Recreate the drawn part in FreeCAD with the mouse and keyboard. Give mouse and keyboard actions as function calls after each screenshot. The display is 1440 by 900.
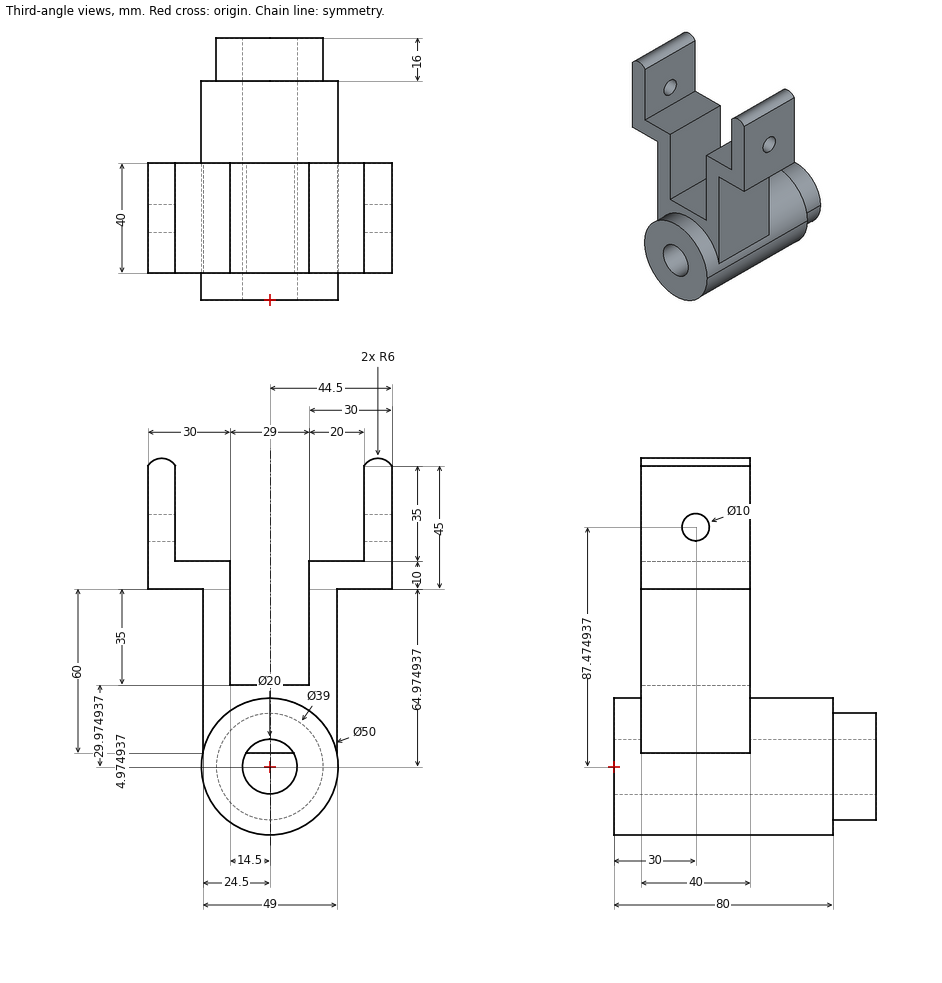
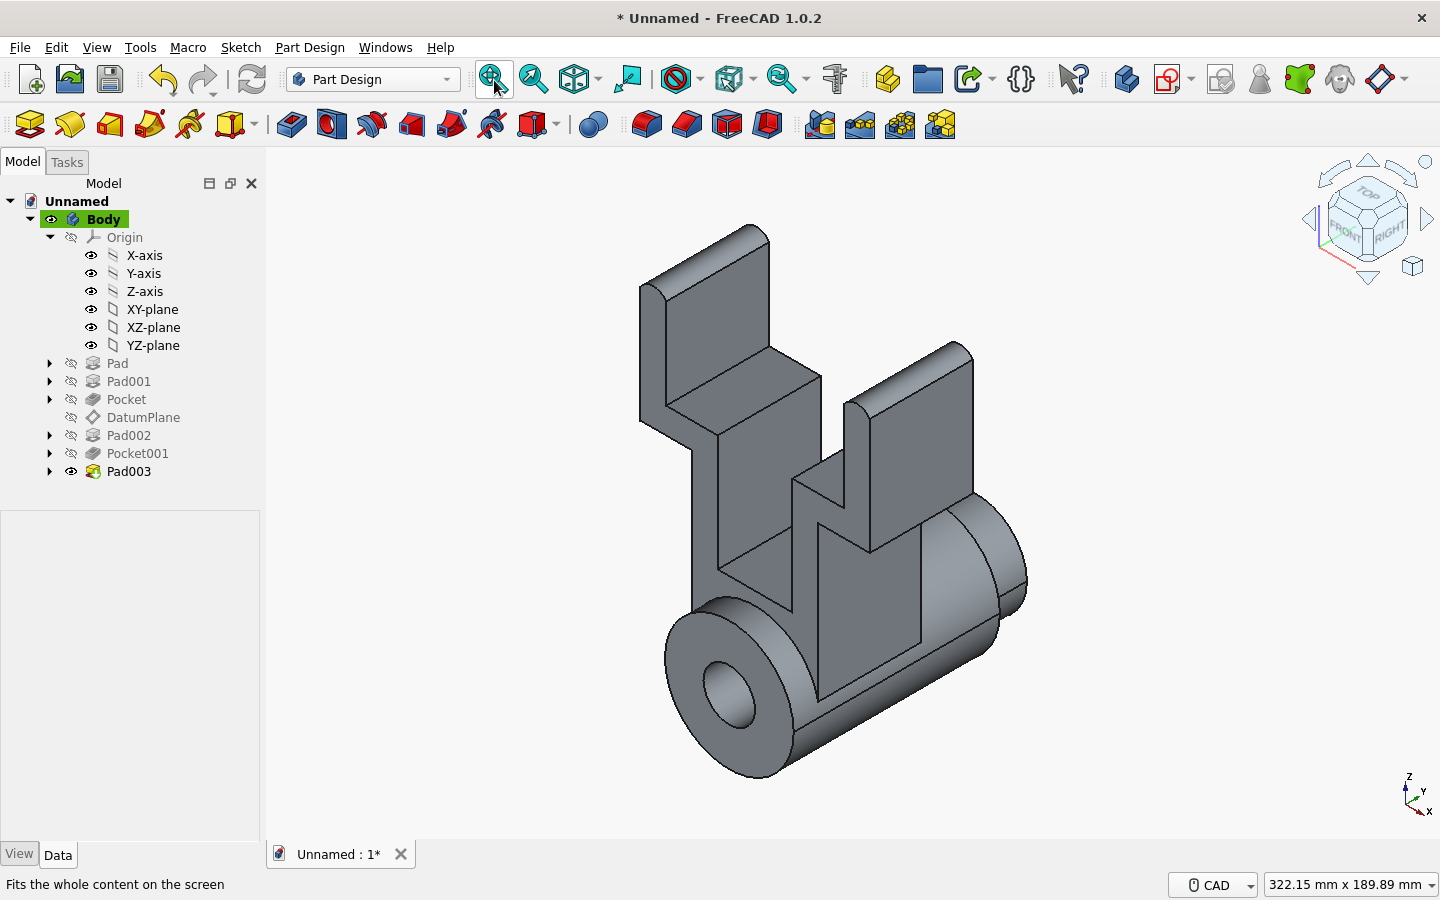
click(921, 455)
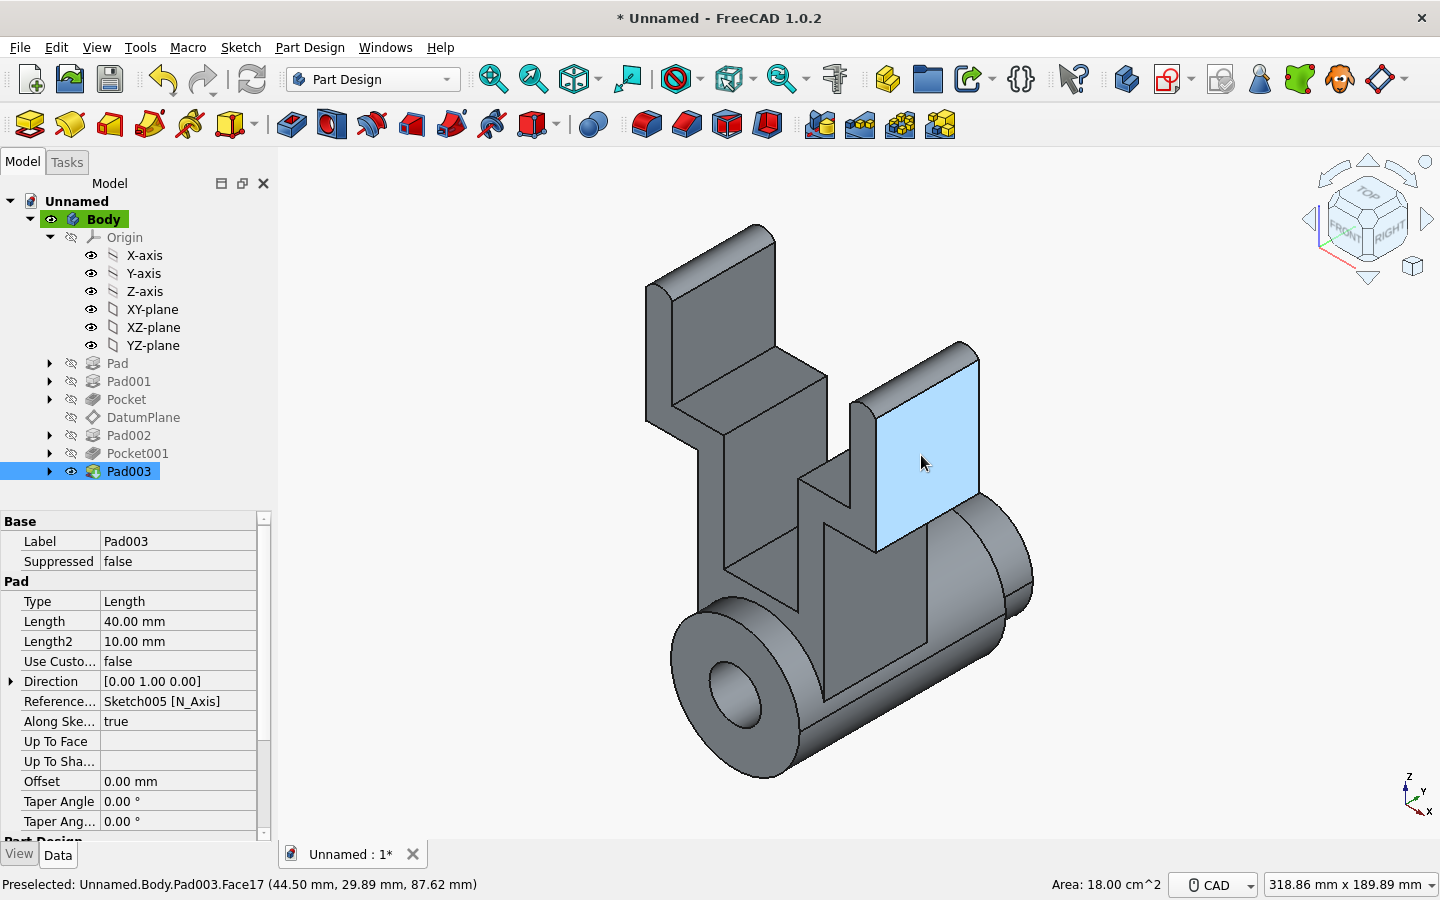
click(1168, 80)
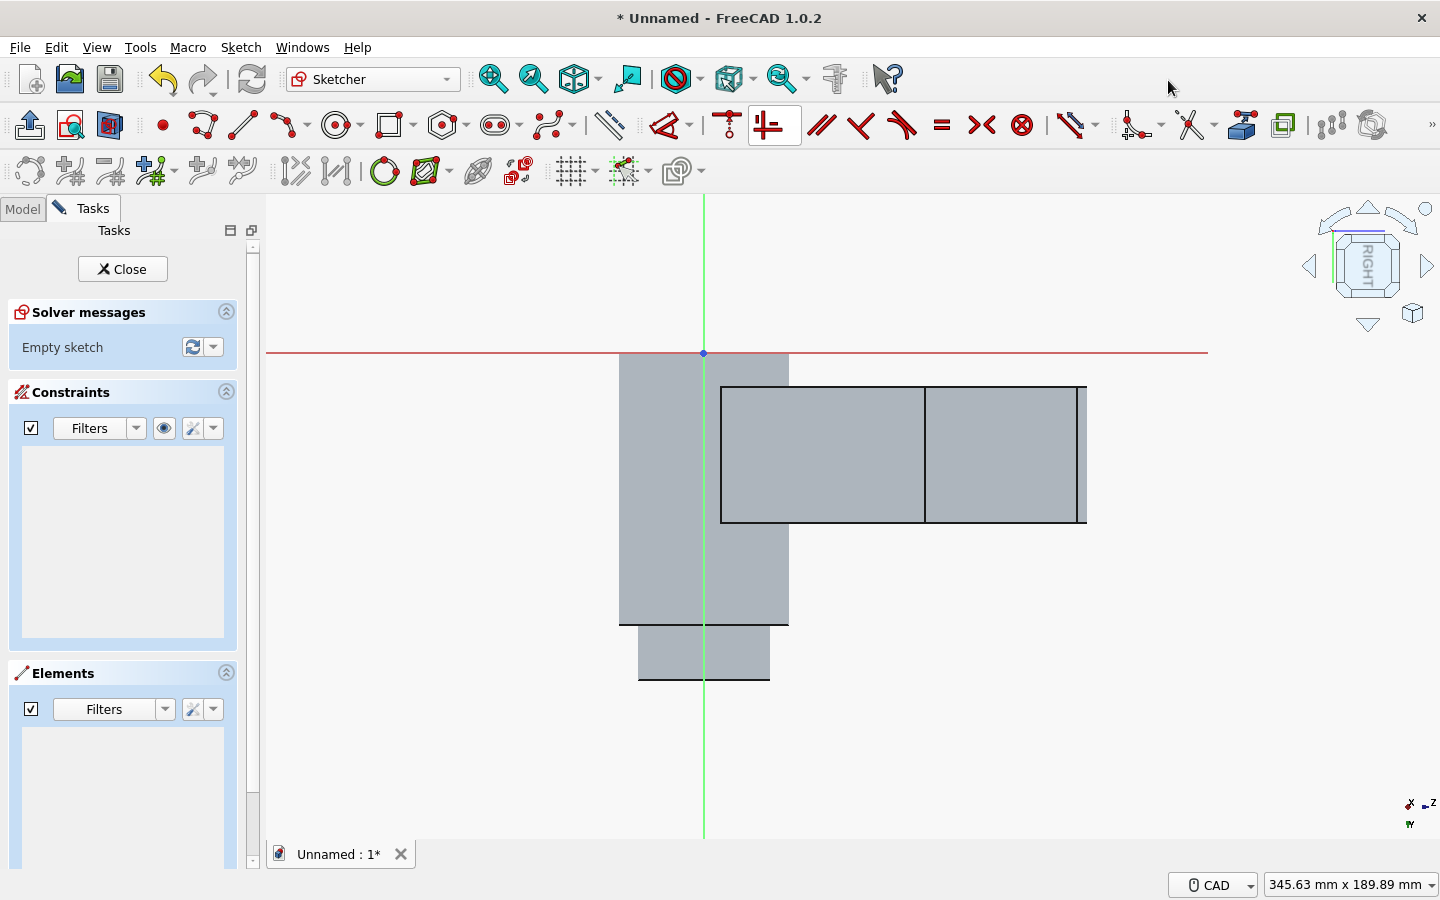
scroll(1018, 450, up, 13)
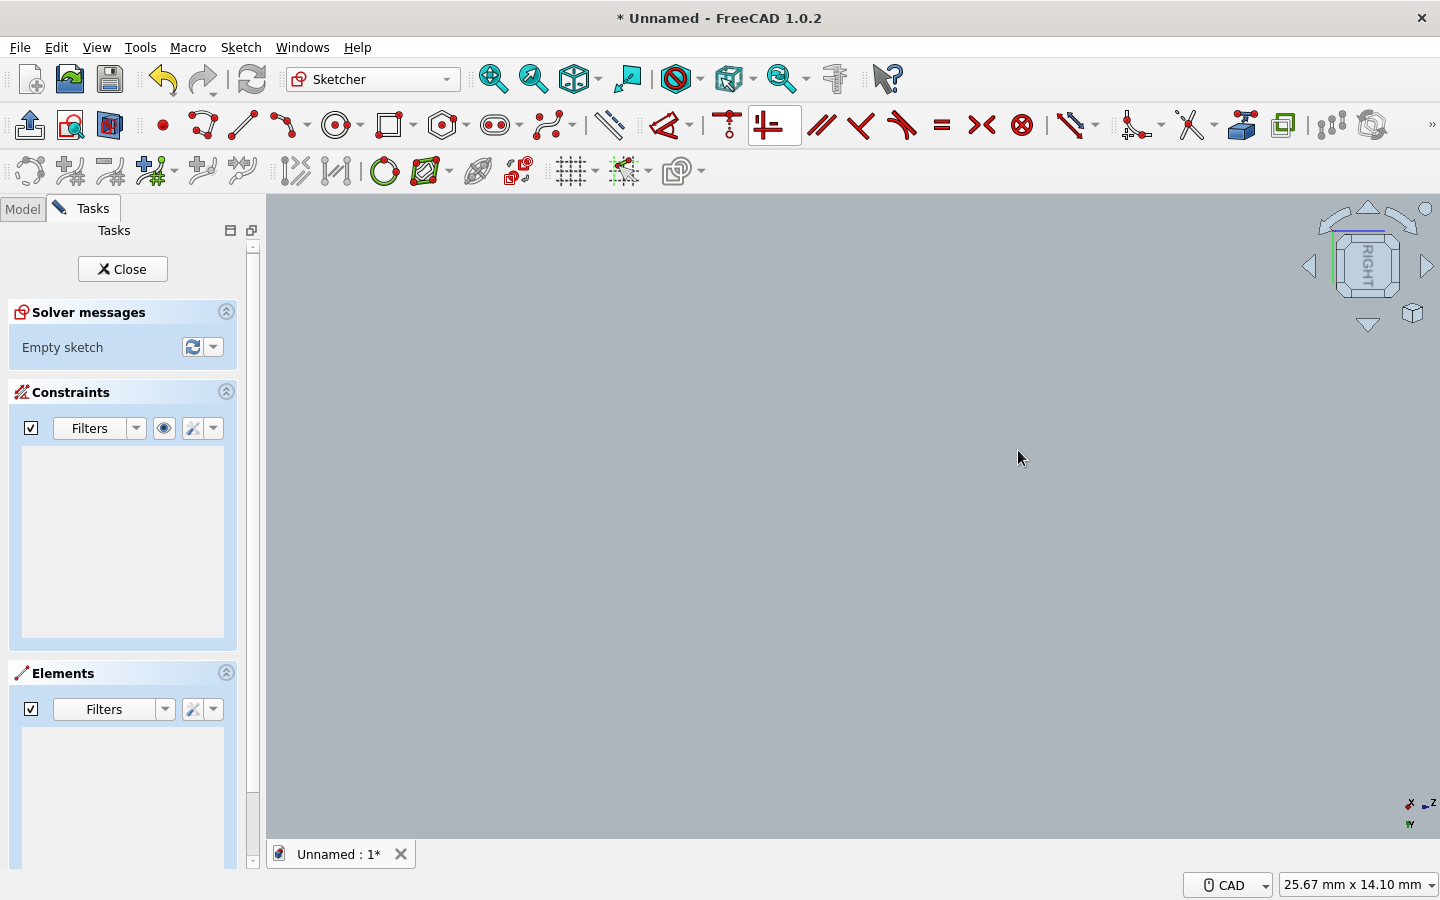
click(336, 126)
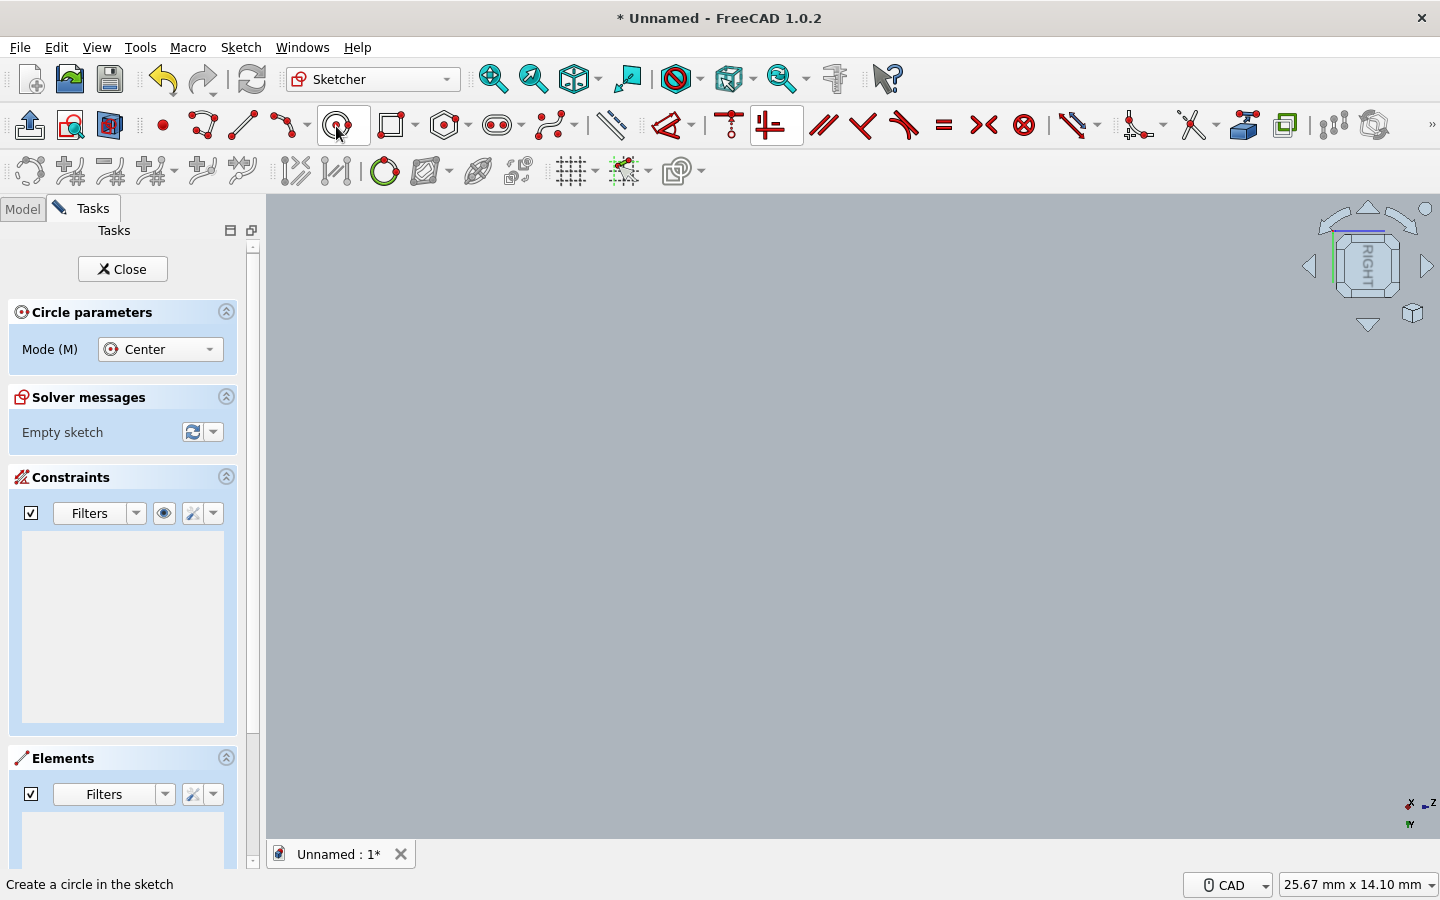
click(782, 517)
click(944, 356)
key(Escape)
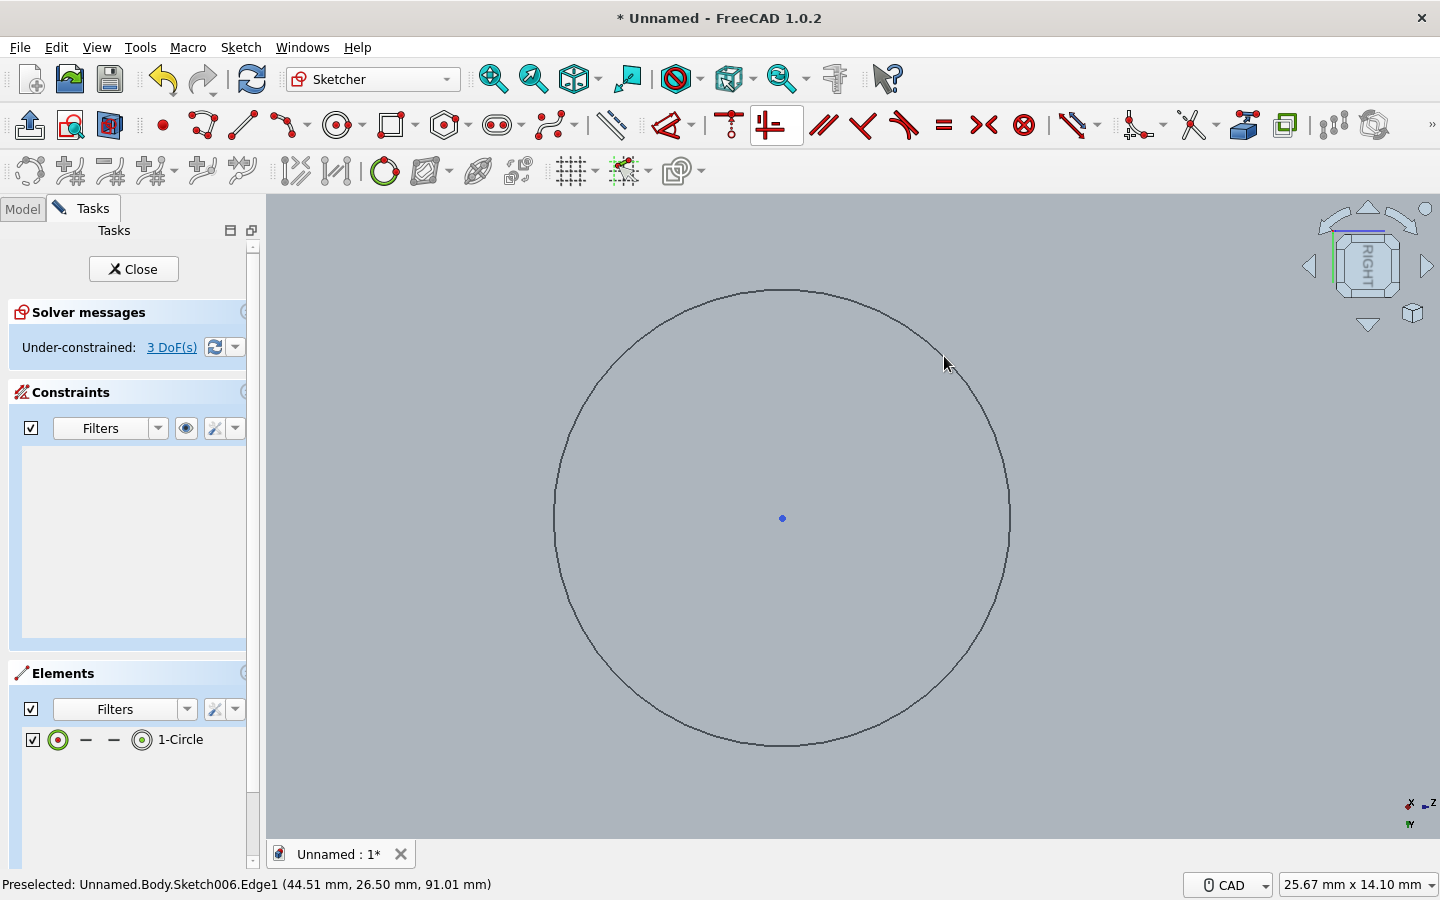
key(d)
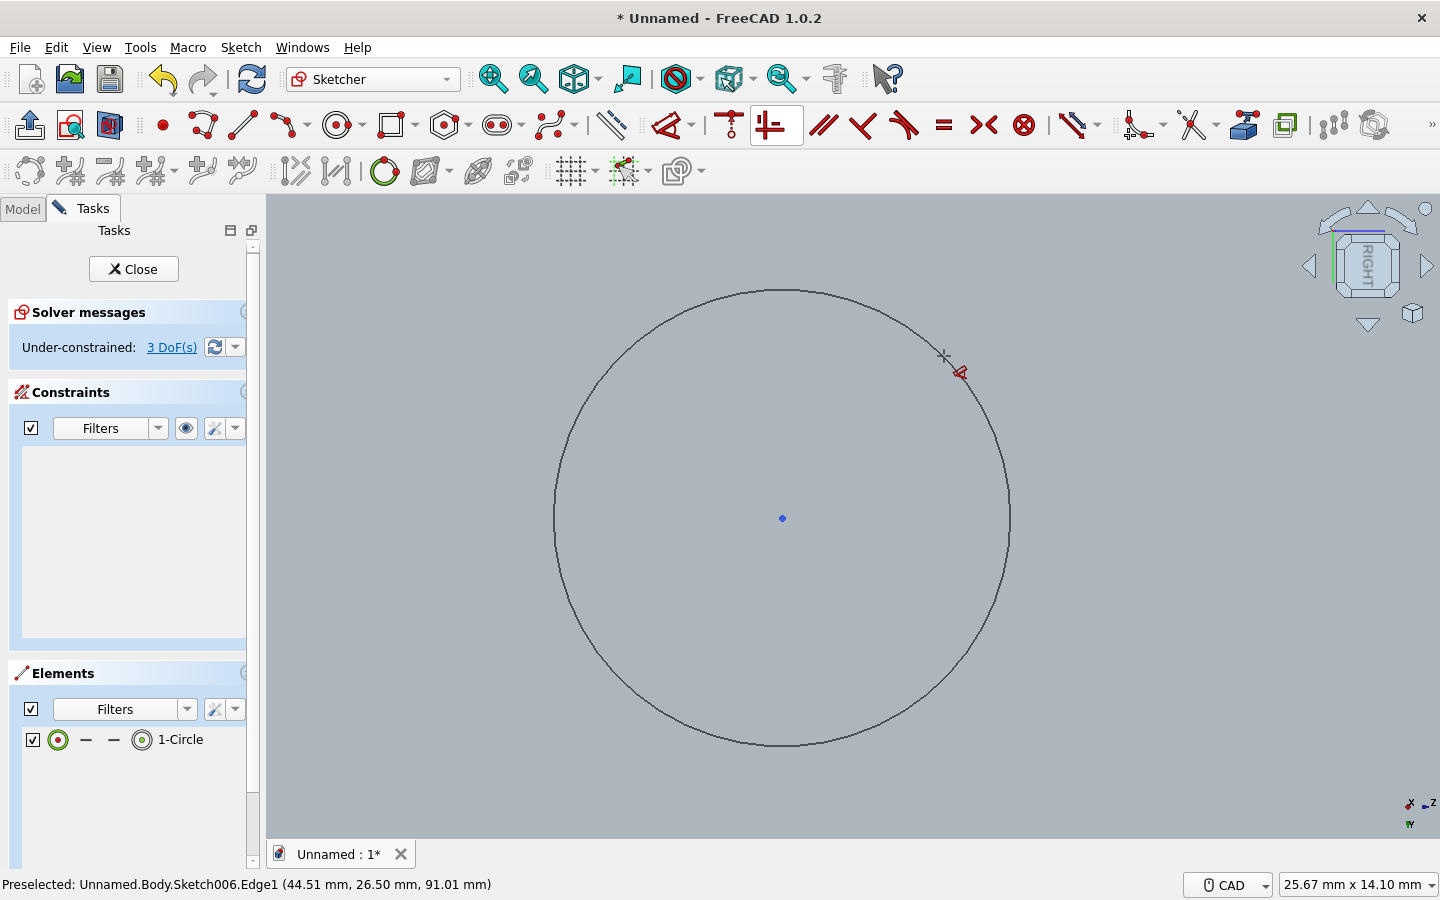
click(943, 356)
click(966, 333)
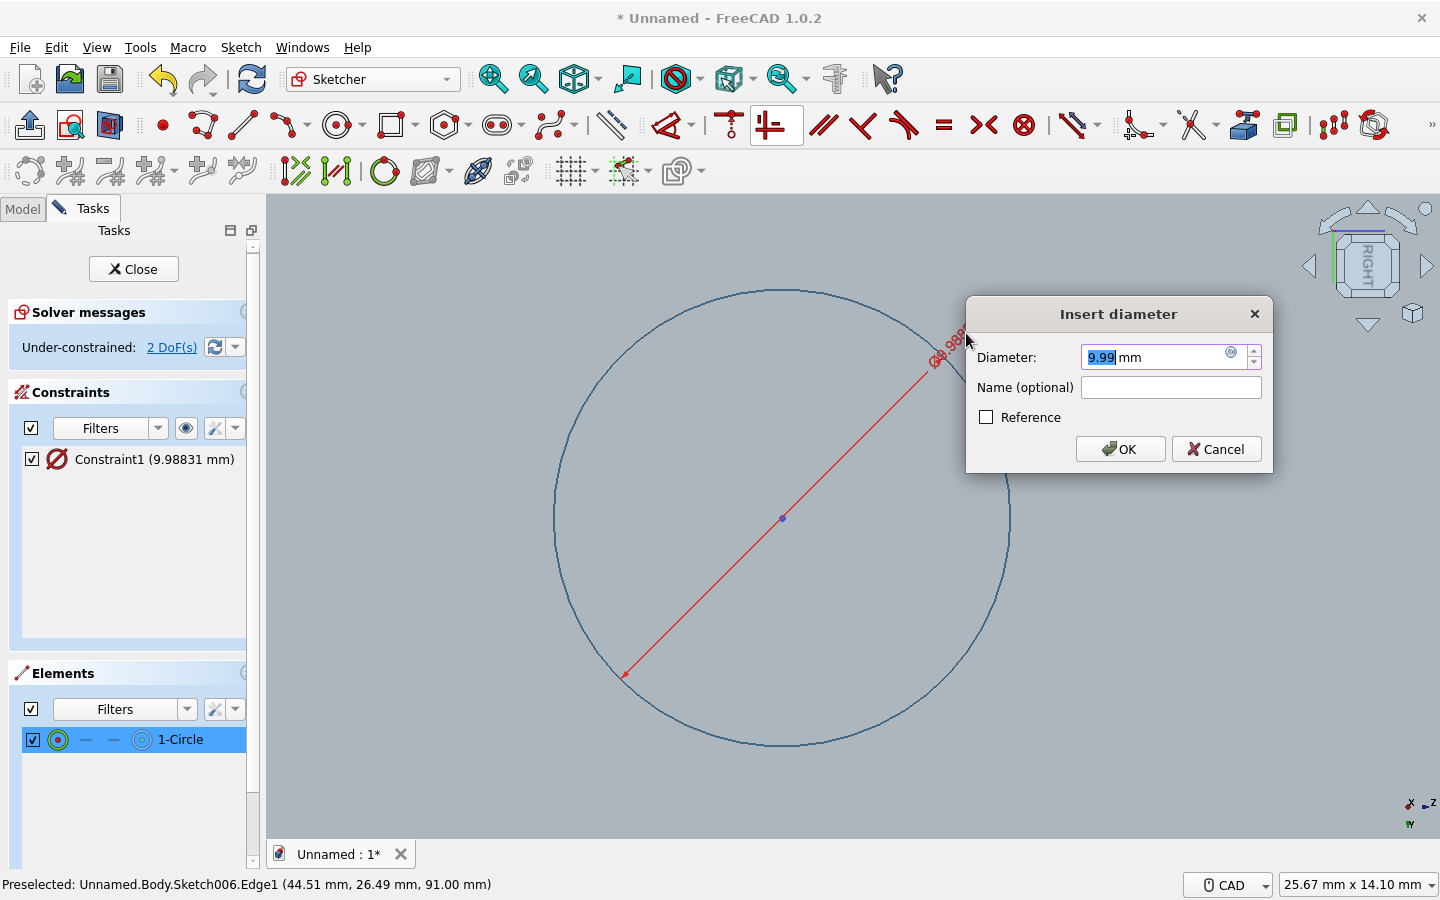
text(10)
key(Return)